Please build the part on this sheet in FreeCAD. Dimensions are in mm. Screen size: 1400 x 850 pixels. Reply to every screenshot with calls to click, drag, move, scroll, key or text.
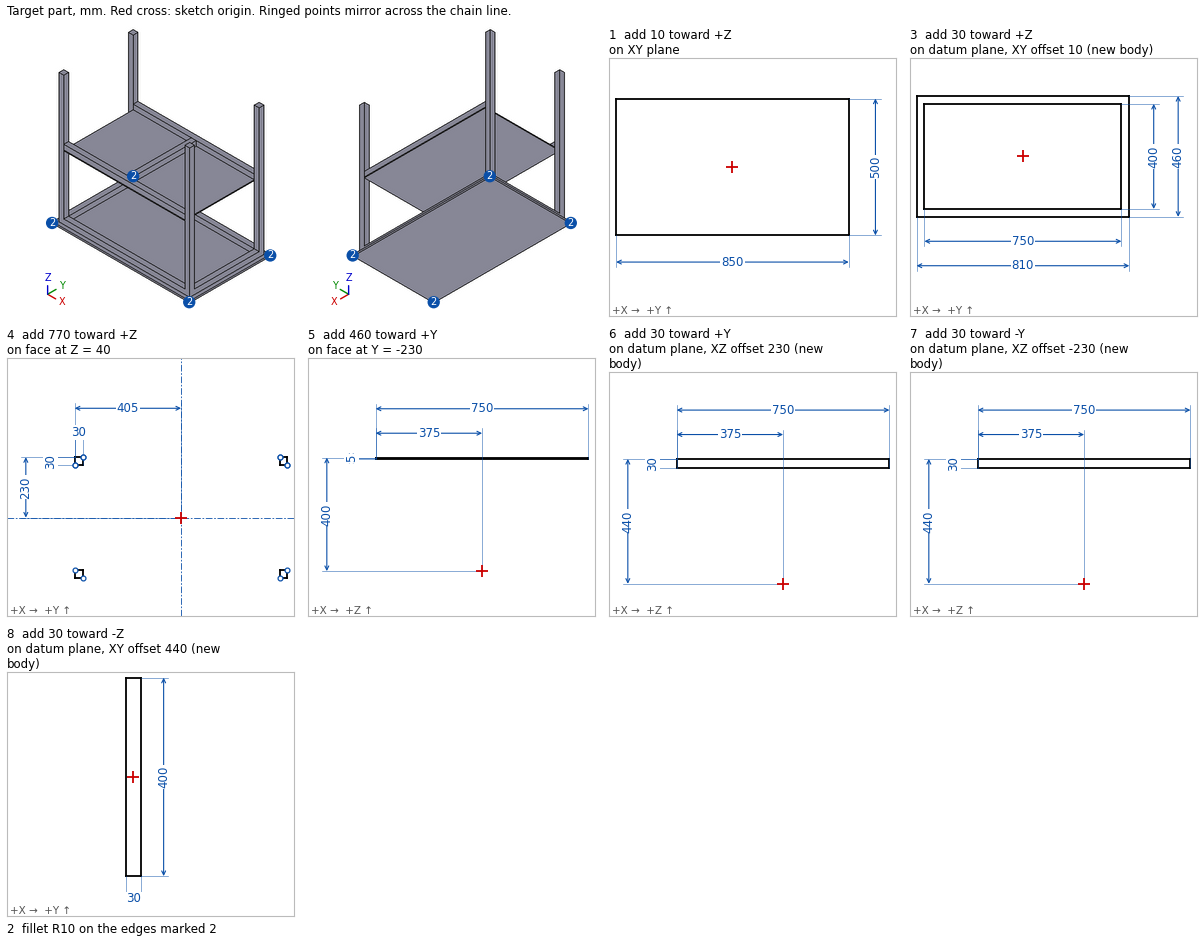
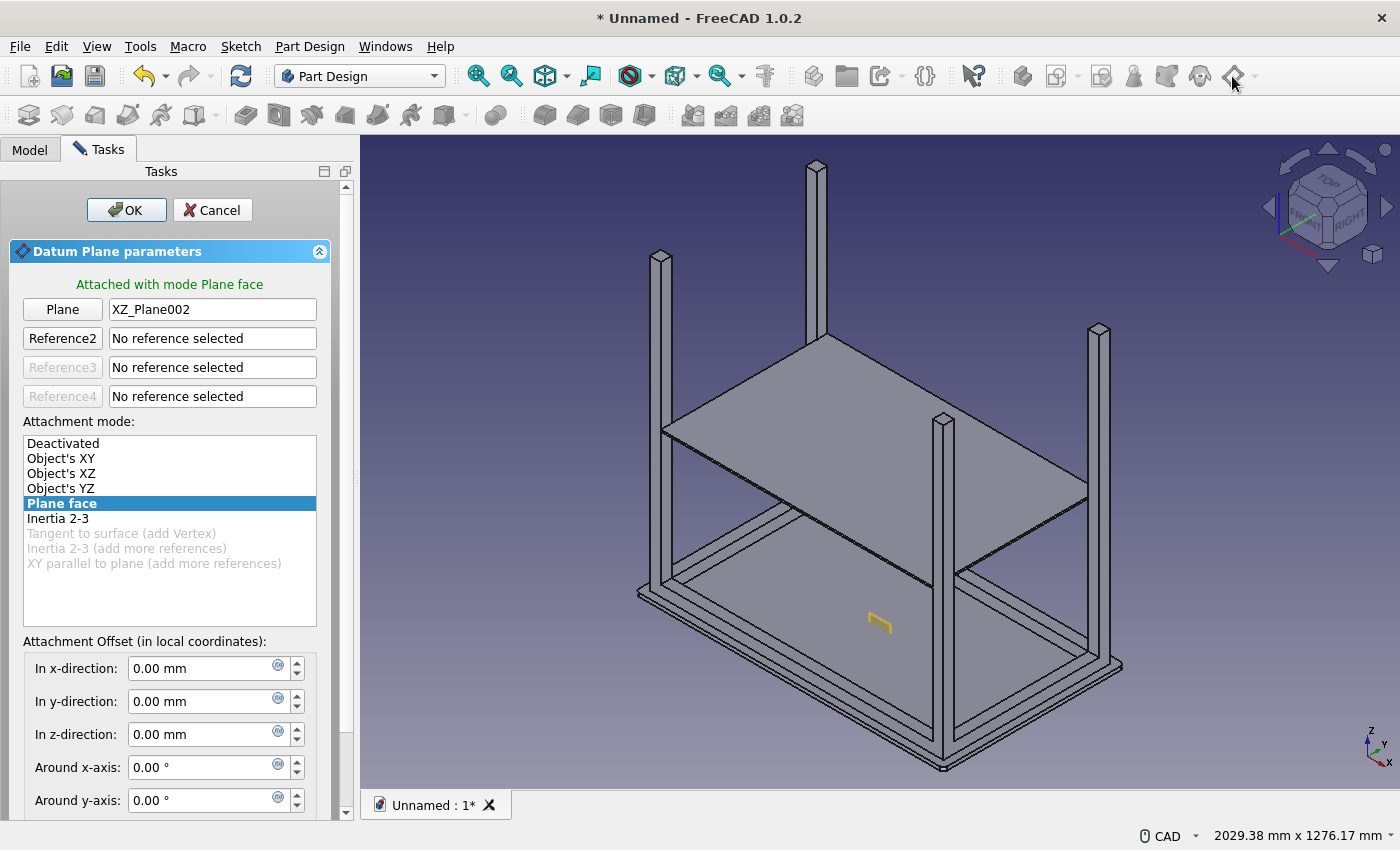
triple_click(210, 734)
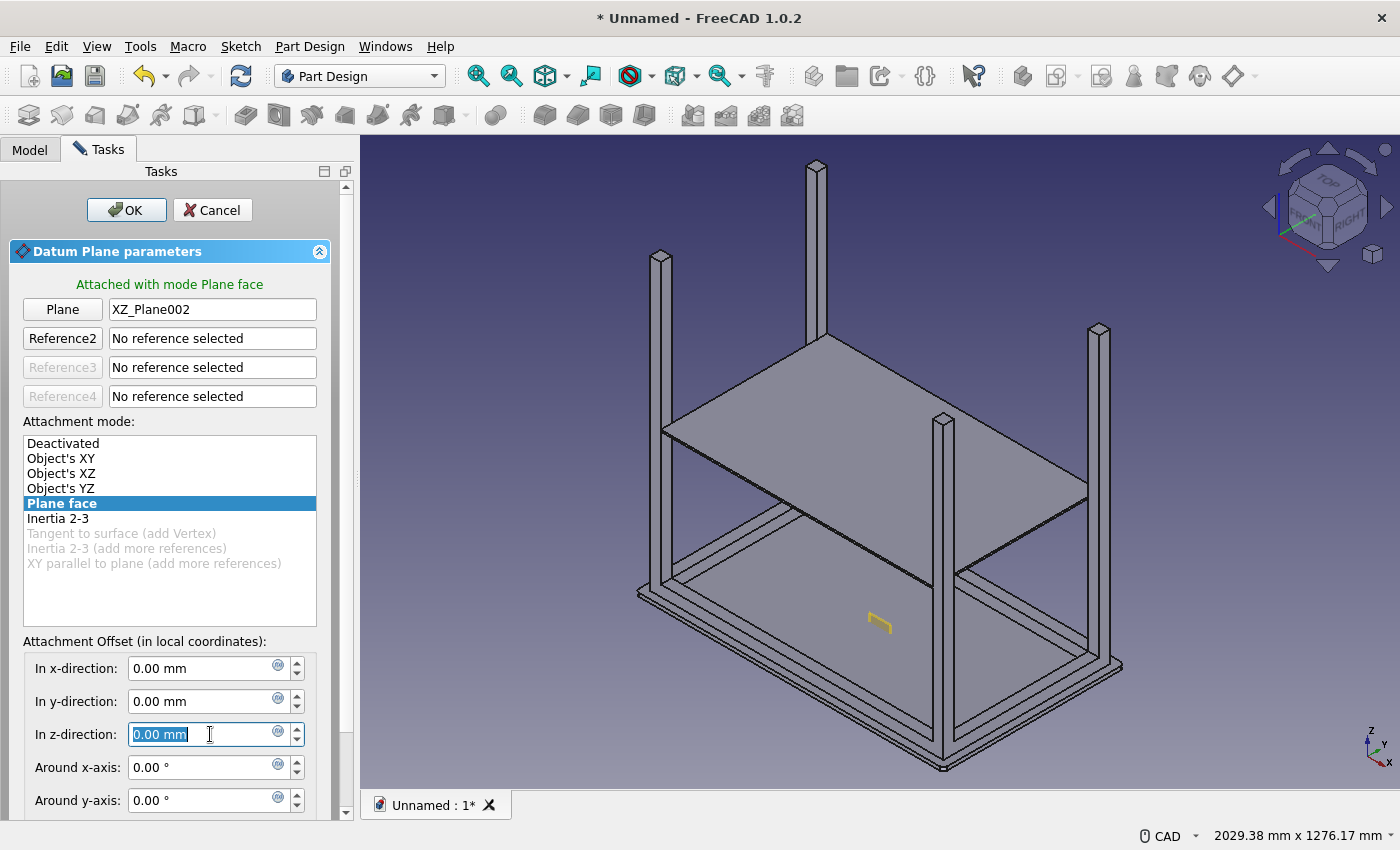
text(230)
key(Tab)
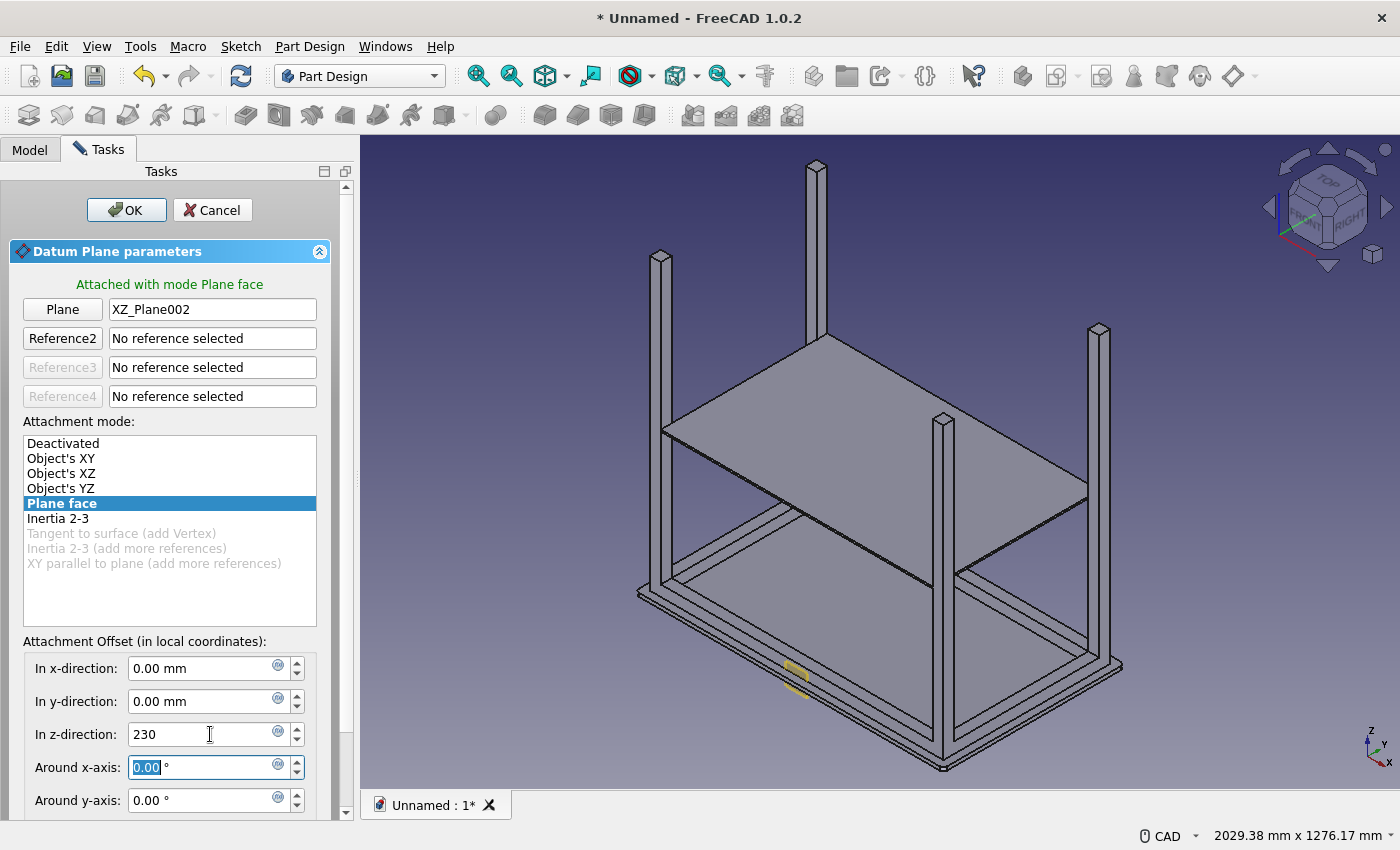
click(127, 210)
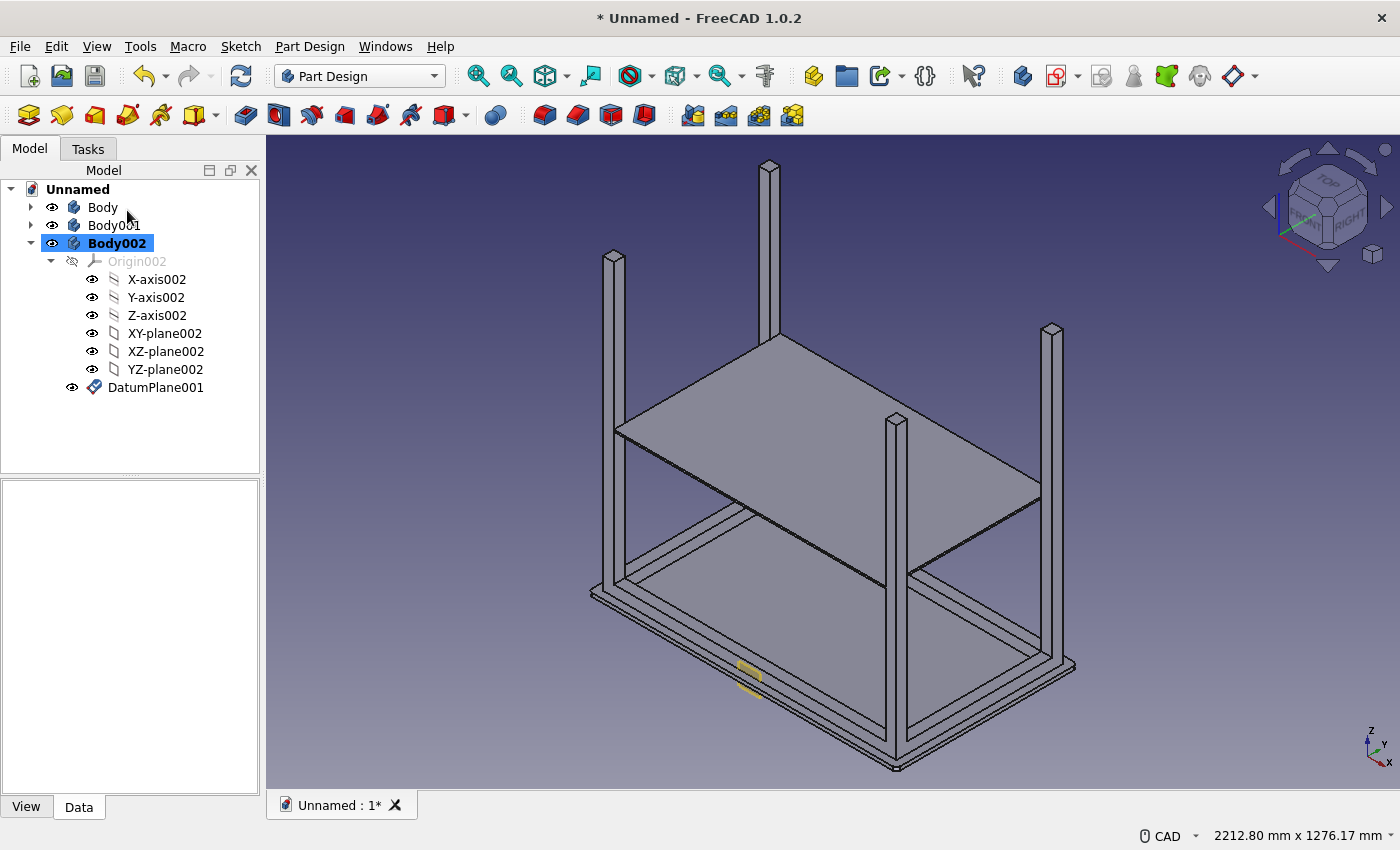
click(117, 387)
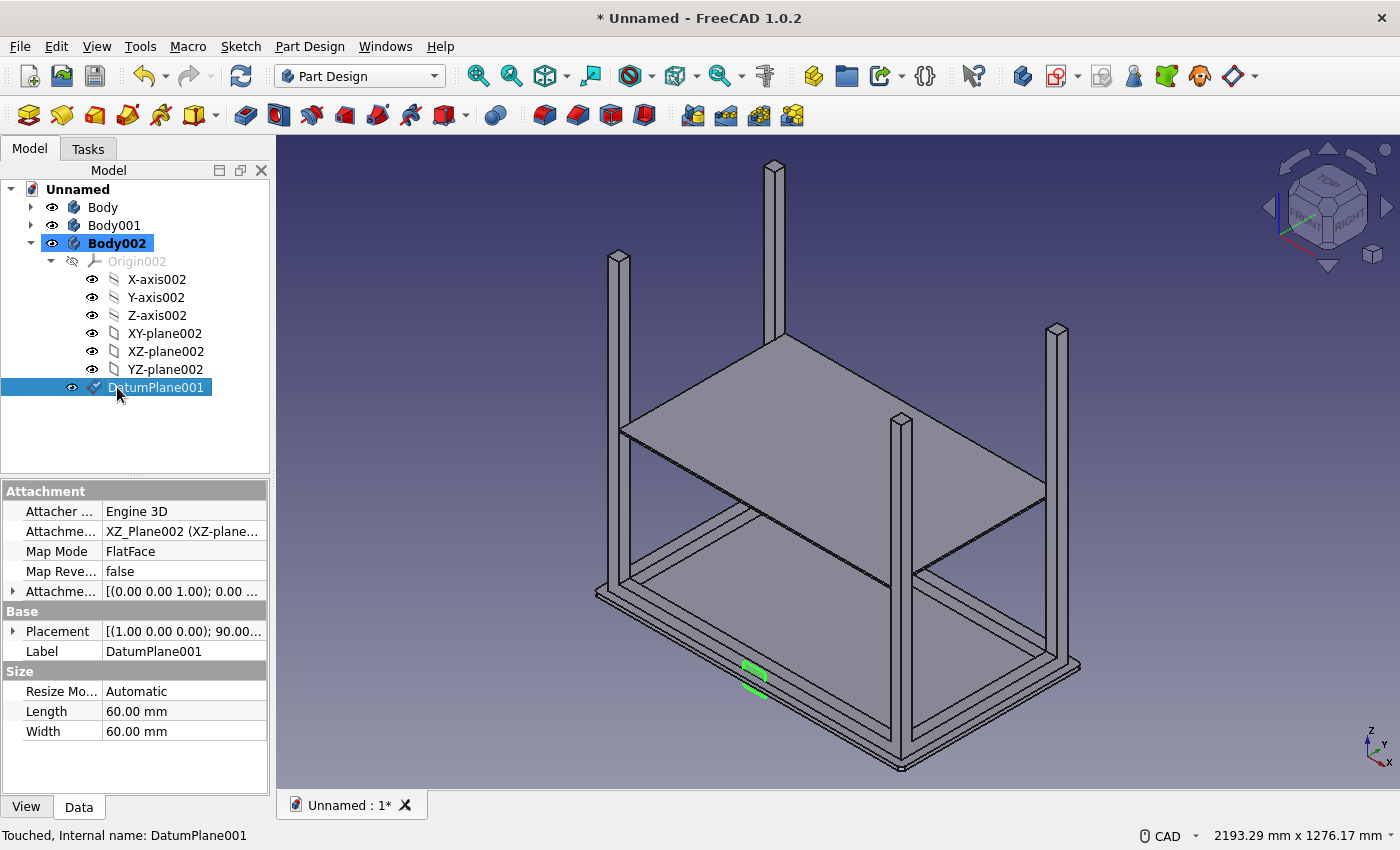
click(1056, 76)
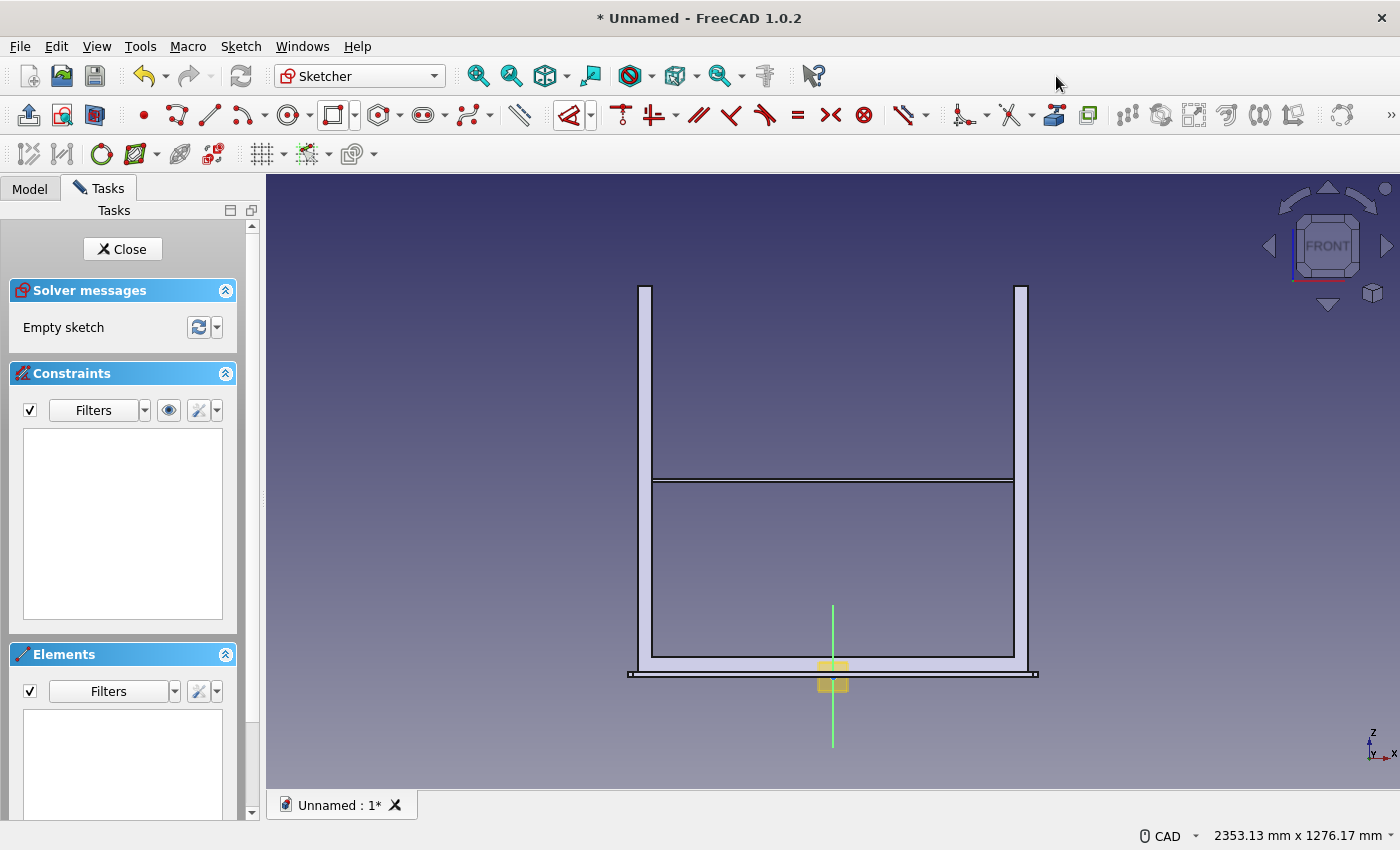
scroll(916, 679, up, 3)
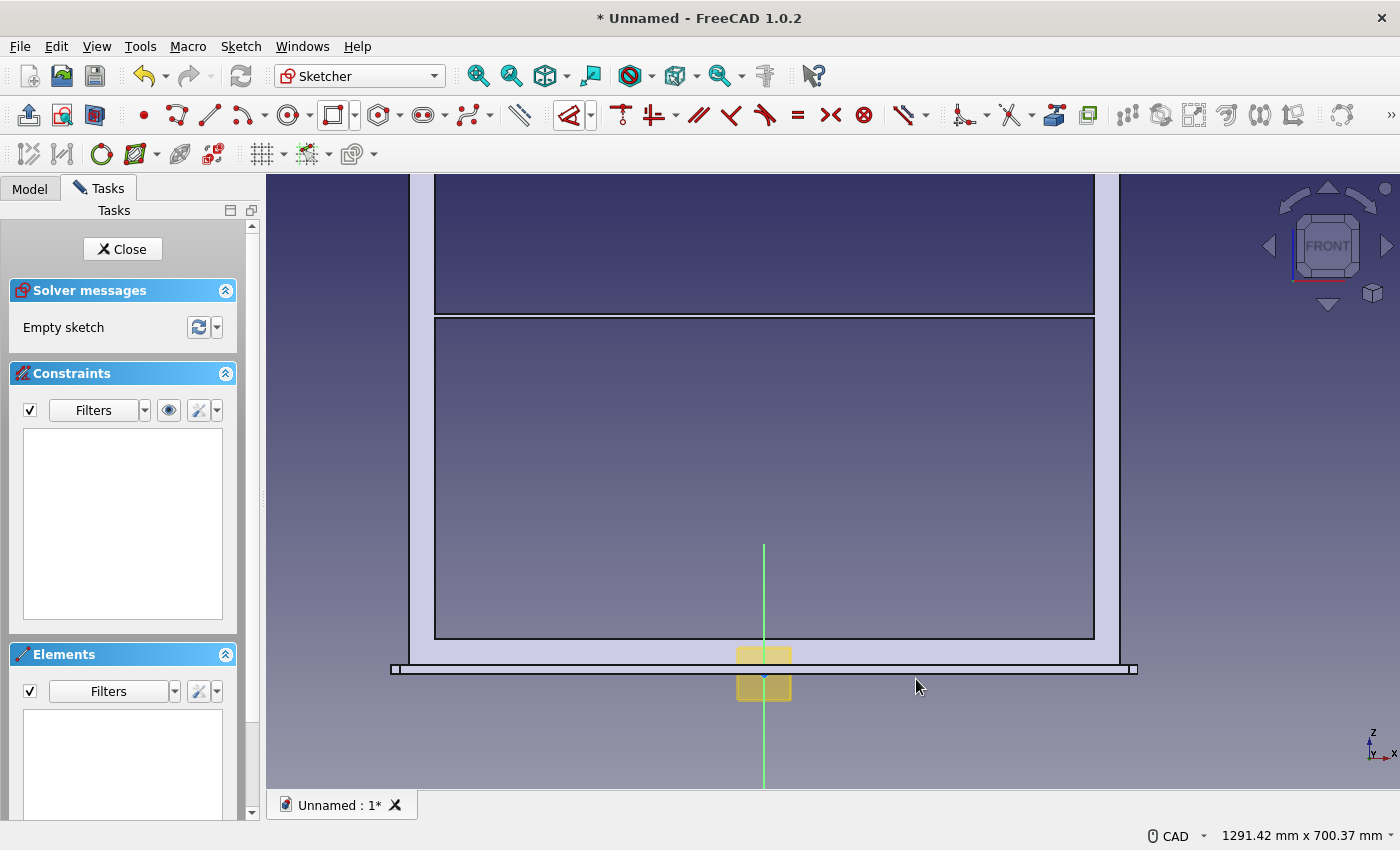
click(332, 116)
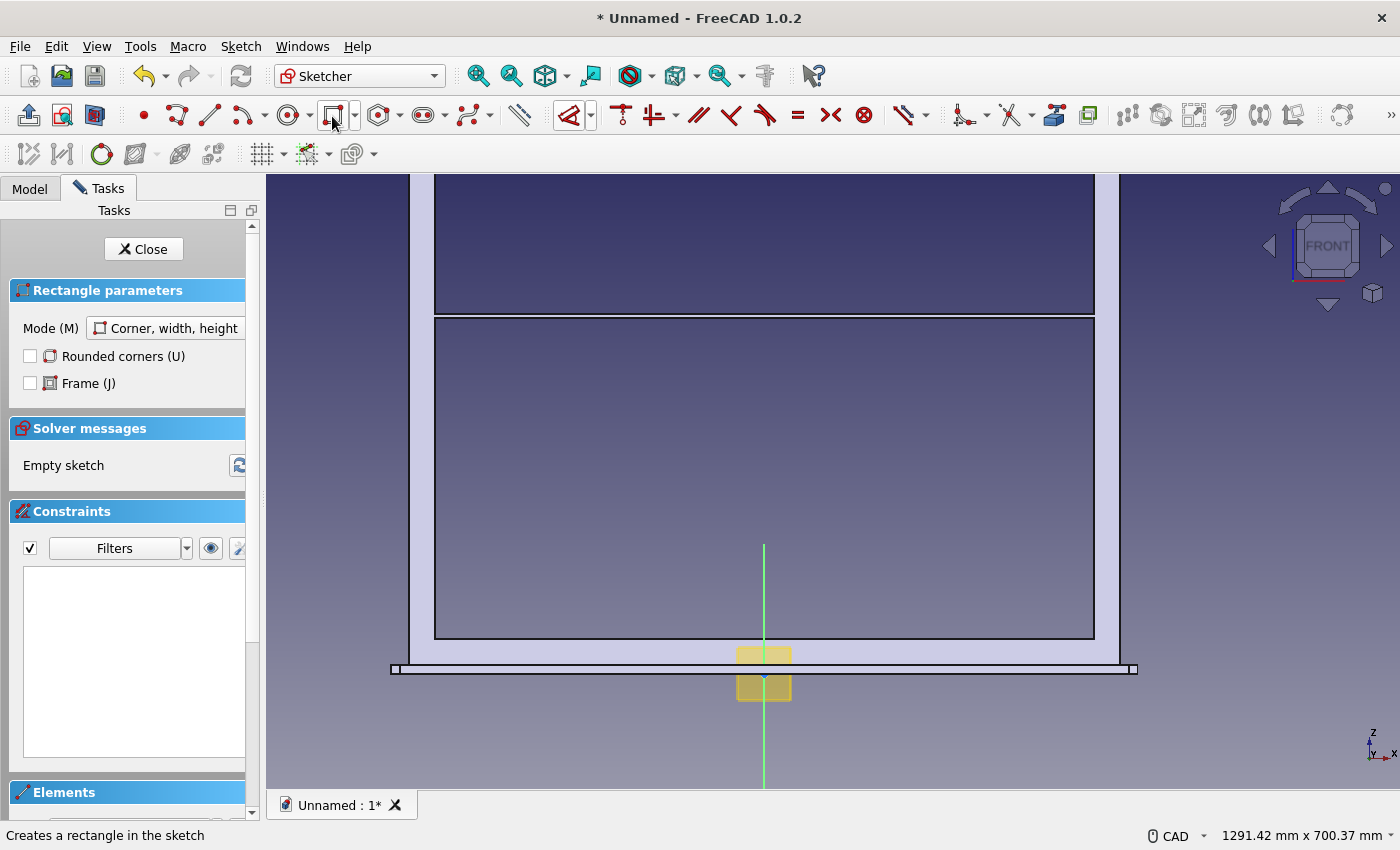
click(435, 288)
click(1094, 314)
key(Escape)